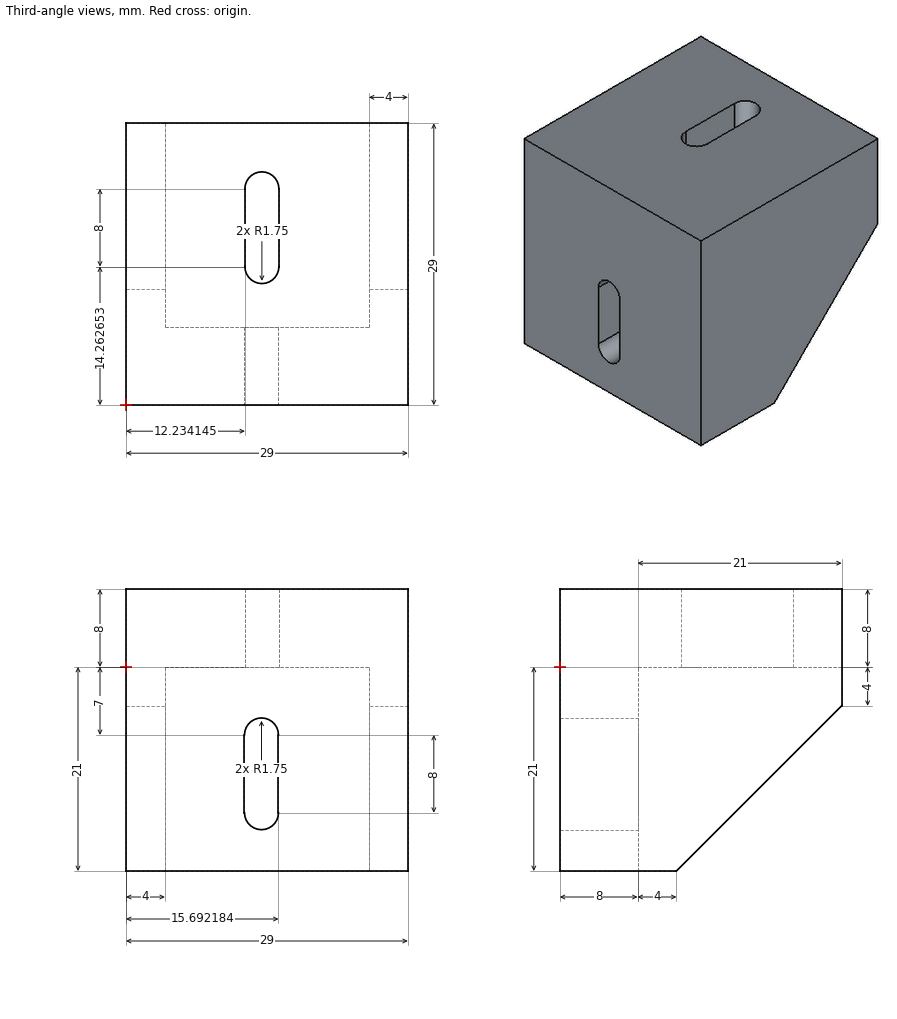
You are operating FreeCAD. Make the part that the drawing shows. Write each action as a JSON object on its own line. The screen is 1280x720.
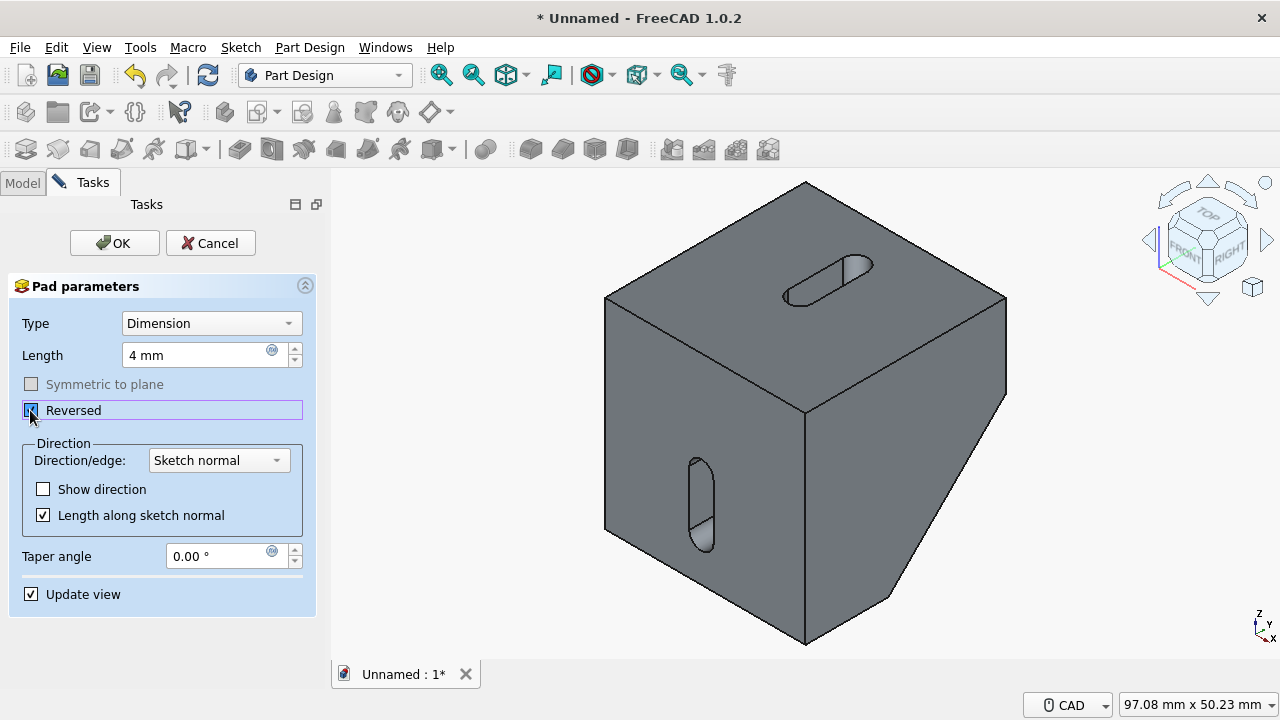
{"action": "left_click", "coordinate": [115, 243]}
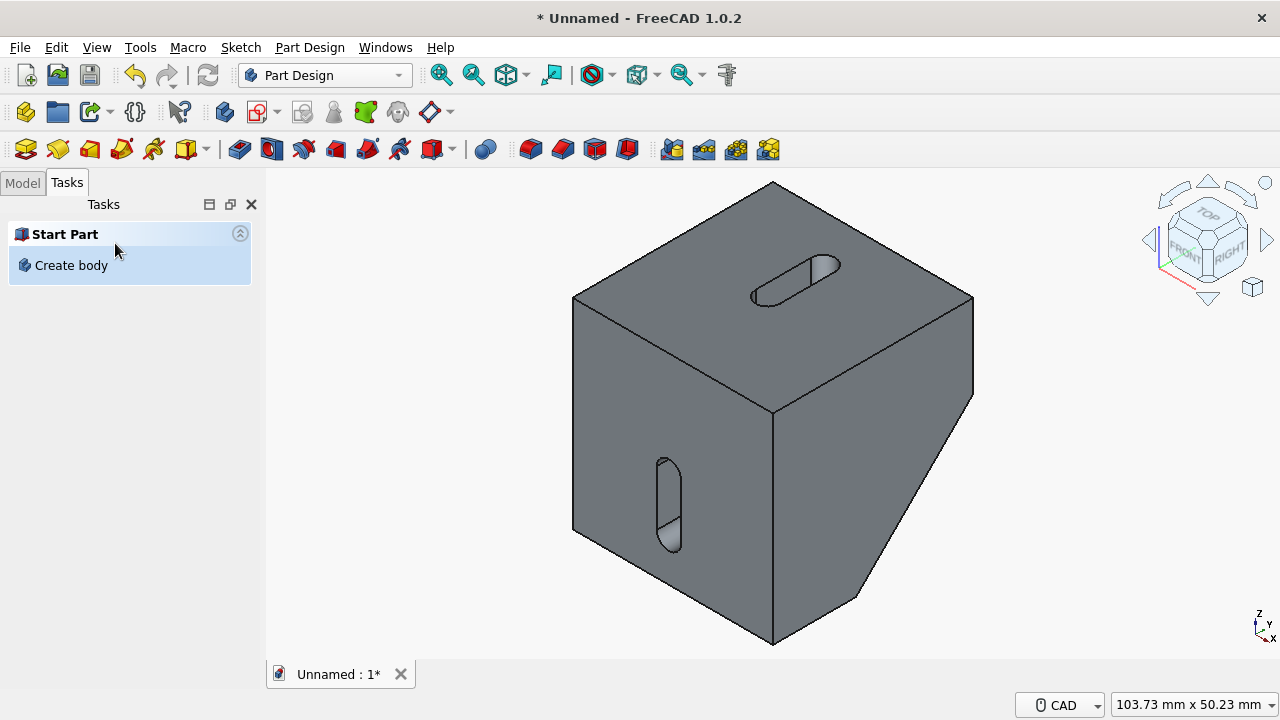
{"action": "key", "text": "6"}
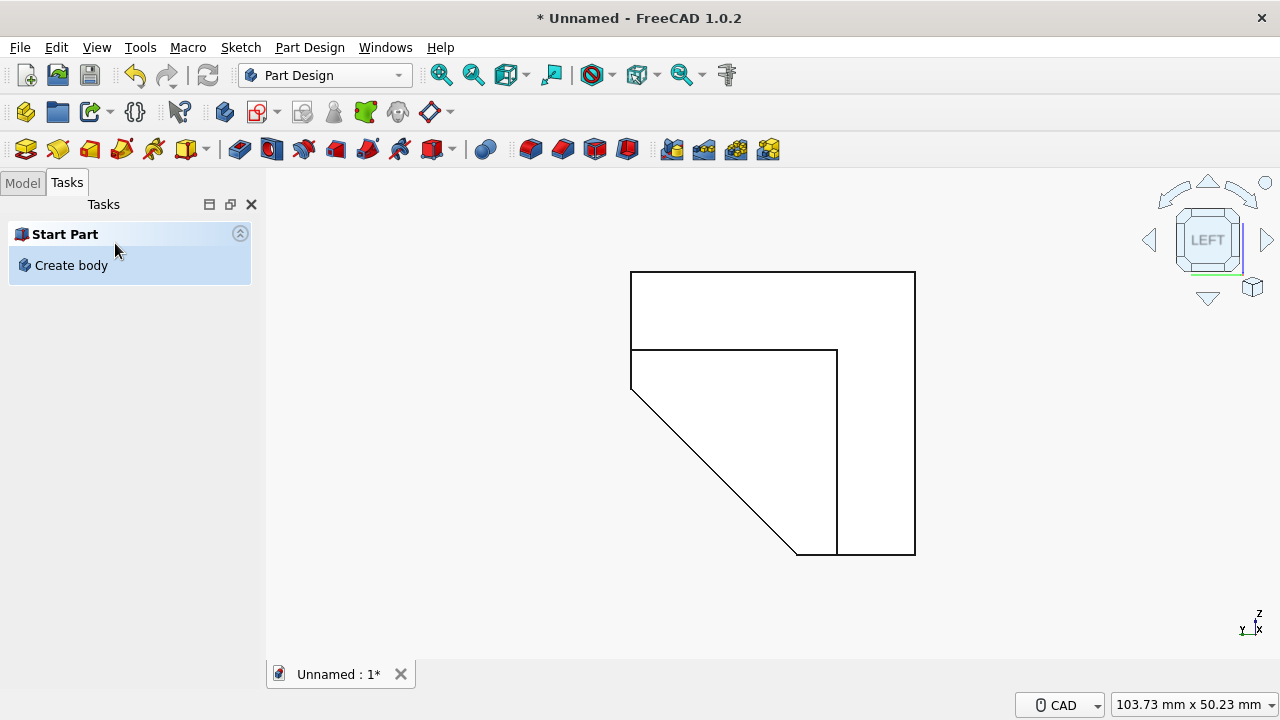
{"action": "left_click", "coordinate": [854, 332]}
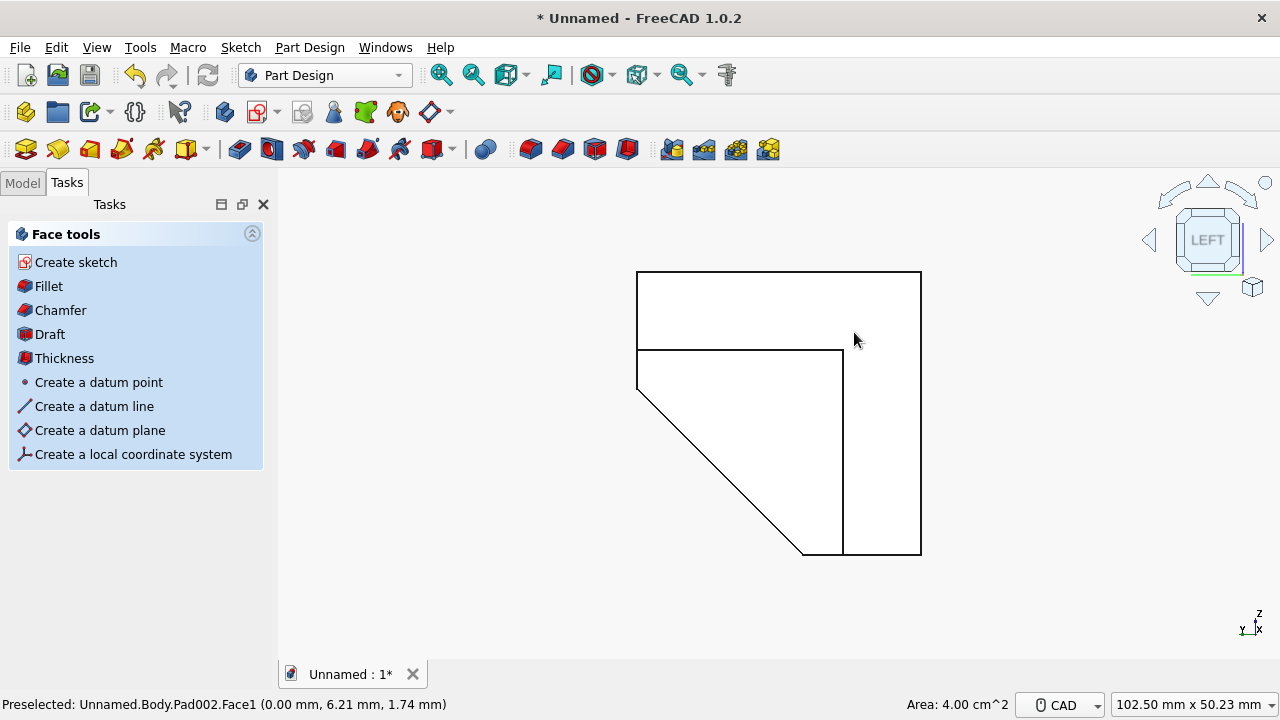
{"action": "left_click", "coordinate": [258, 112]}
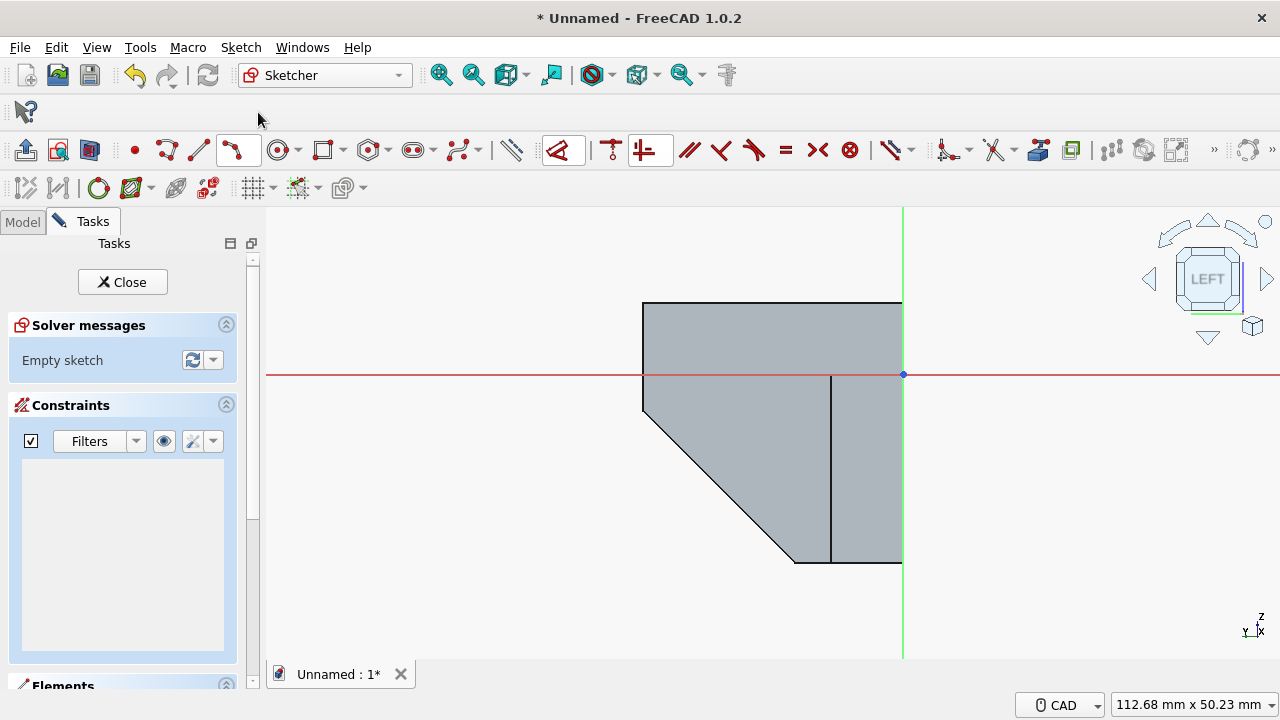
{"action": "scroll", "coordinate": [912, 542], "scroll_direction": "up", "scroll_amount": 2}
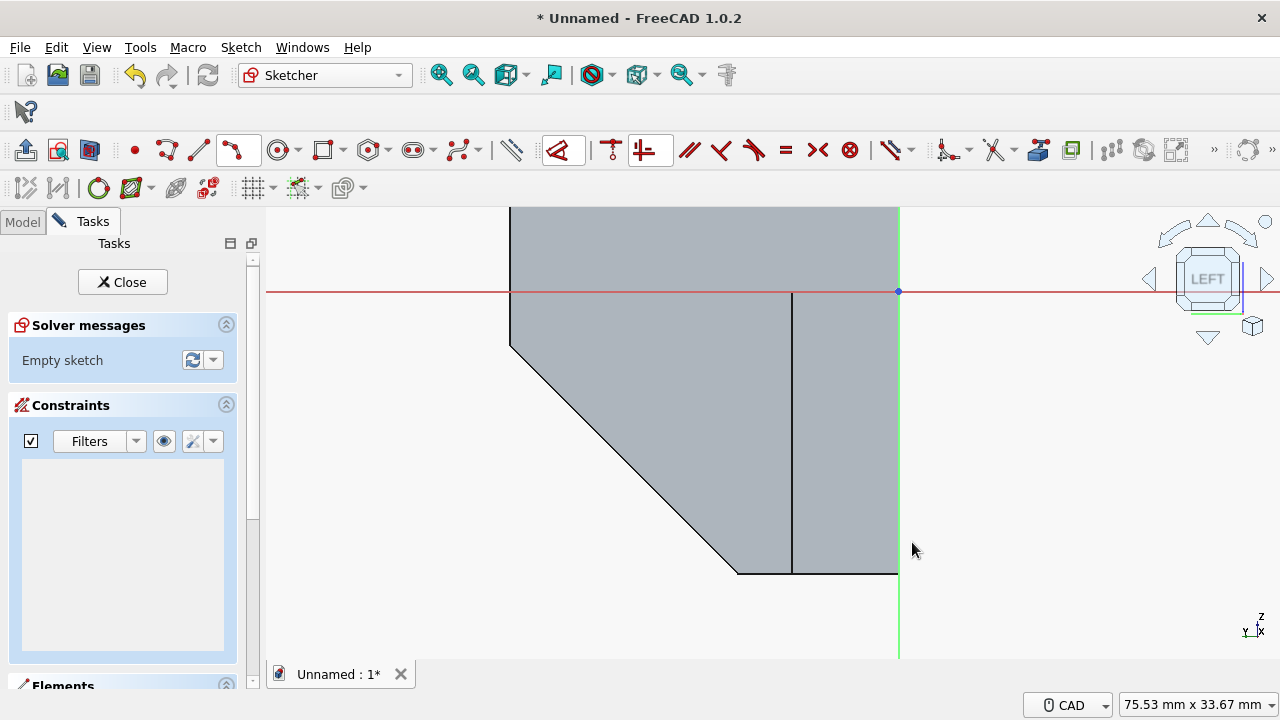
{"action": "left_click", "coordinate": [168, 150]}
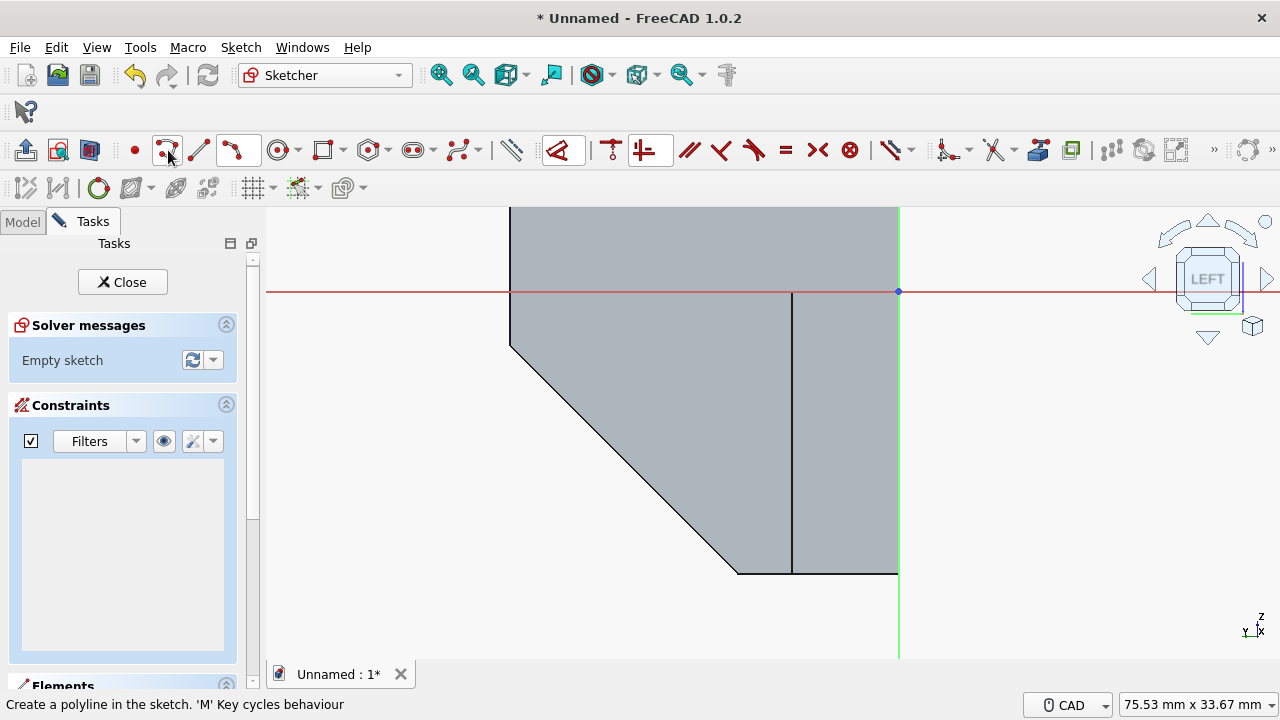
{"action": "left_click", "coordinate": [792, 292]}
{"action": "left_click", "coordinate": [510, 301]}
{"action": "left_click", "coordinate": [510, 345]}
{"action": "left_click", "coordinate": [738, 574]}
{"action": "left_click", "coordinate": [792, 574]}
{"action": "left_click", "coordinate": [792, 292]}
{"action": "key", "text": "Escape"}
{"action": "key", "text": "Escape"}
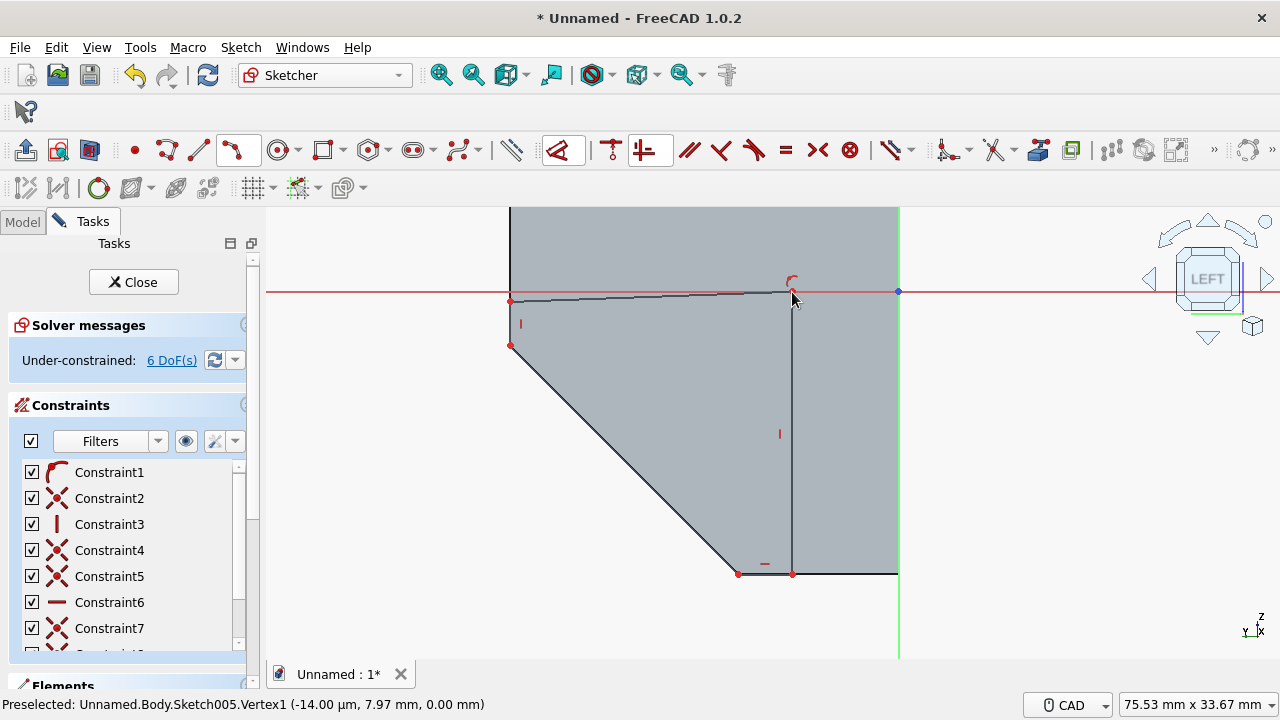
{"action": "left_click", "coordinate": [707, 295]}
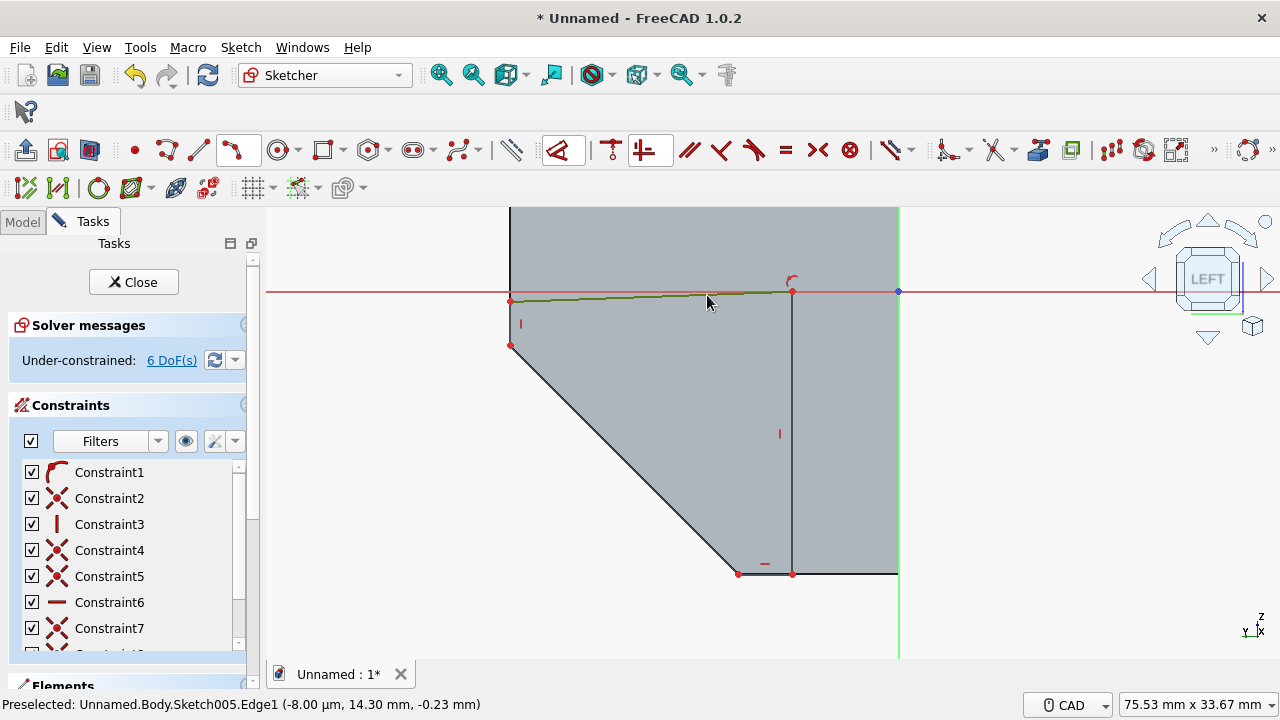
{"action": "left_click", "coordinate": [668, 150]}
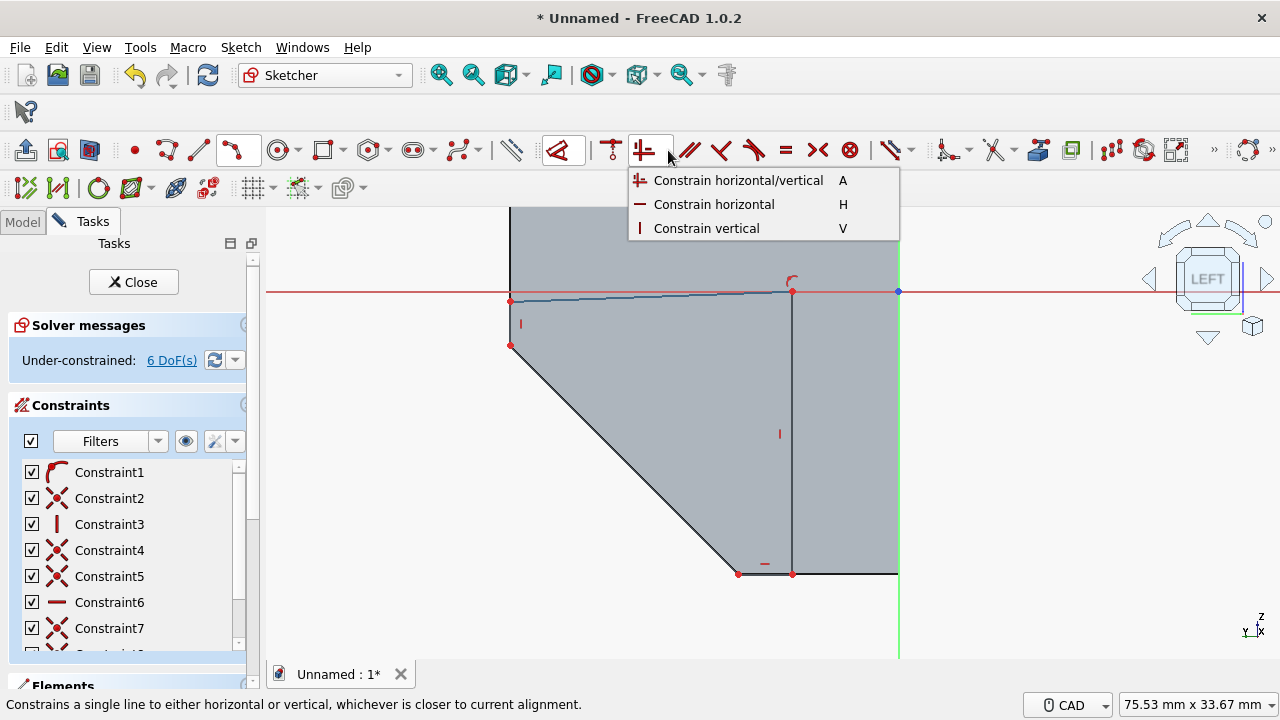
{"action": "left_click", "coordinate": [764, 204]}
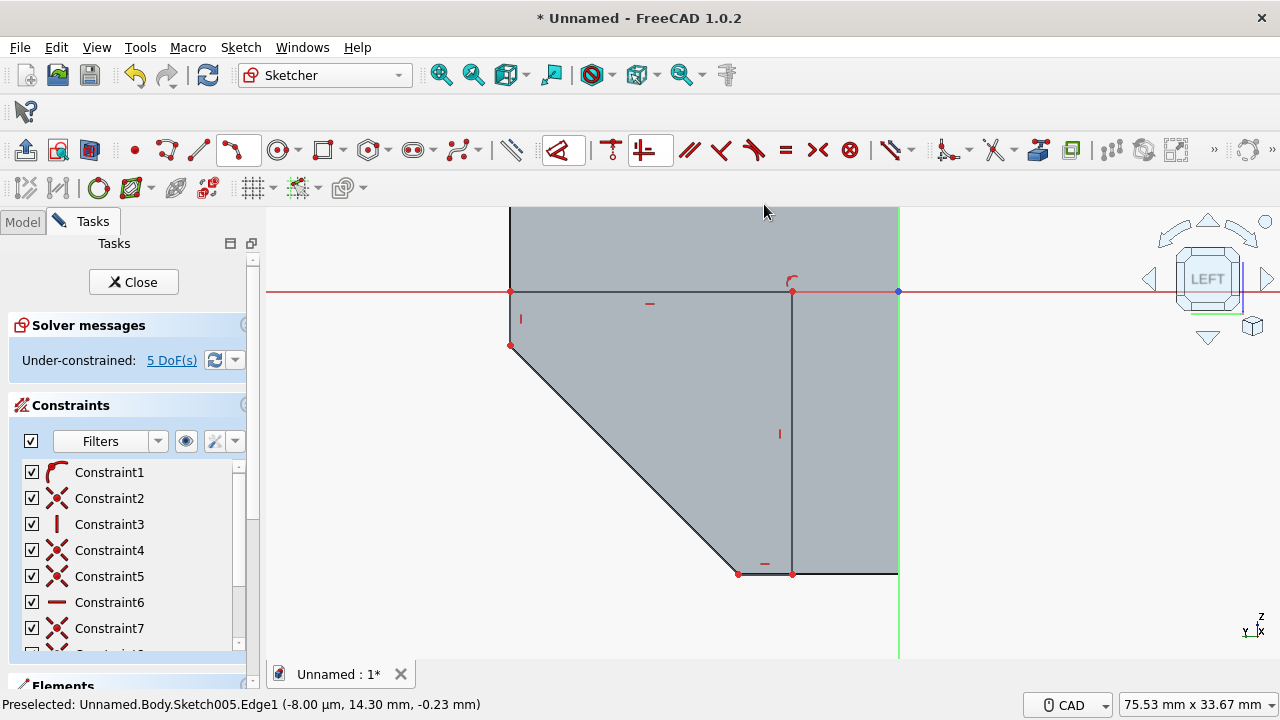
{"action": "left_click", "coordinate": [510, 308]}